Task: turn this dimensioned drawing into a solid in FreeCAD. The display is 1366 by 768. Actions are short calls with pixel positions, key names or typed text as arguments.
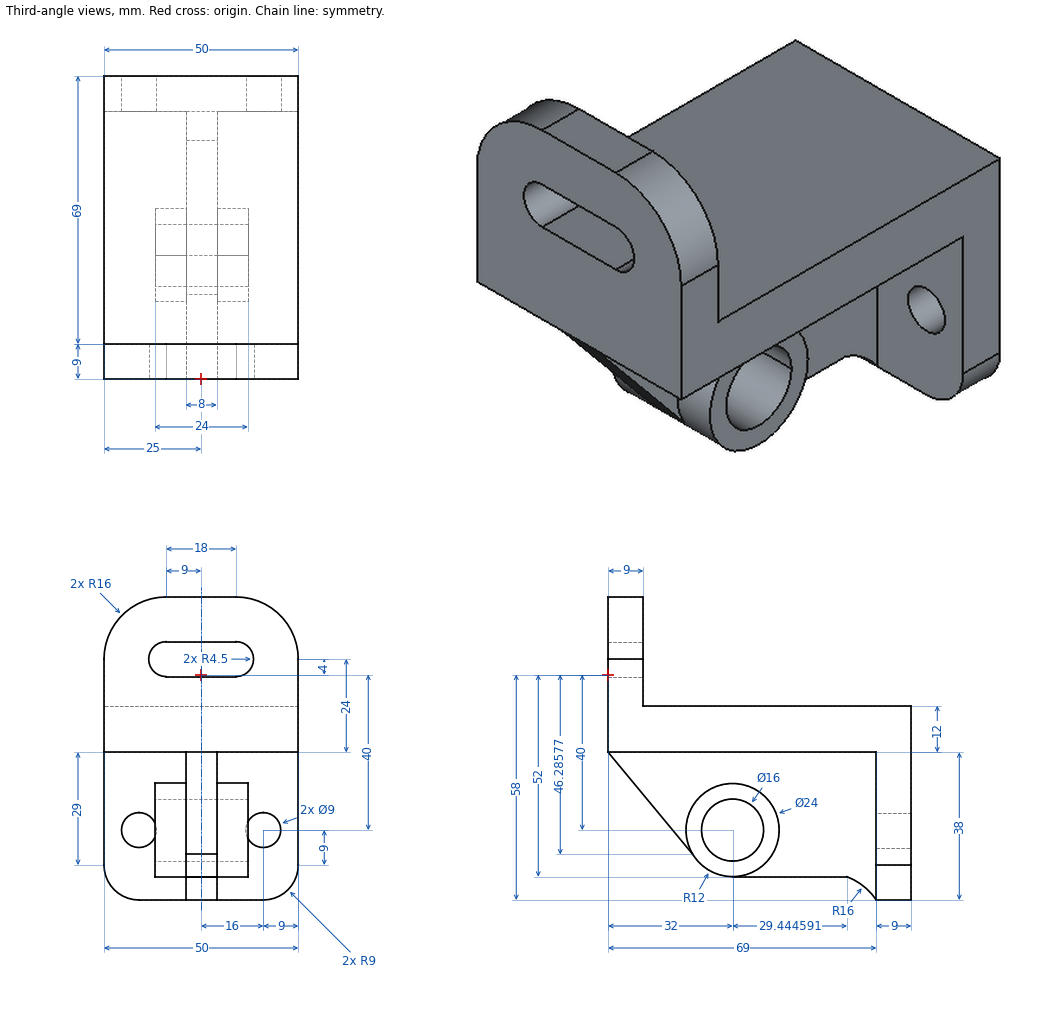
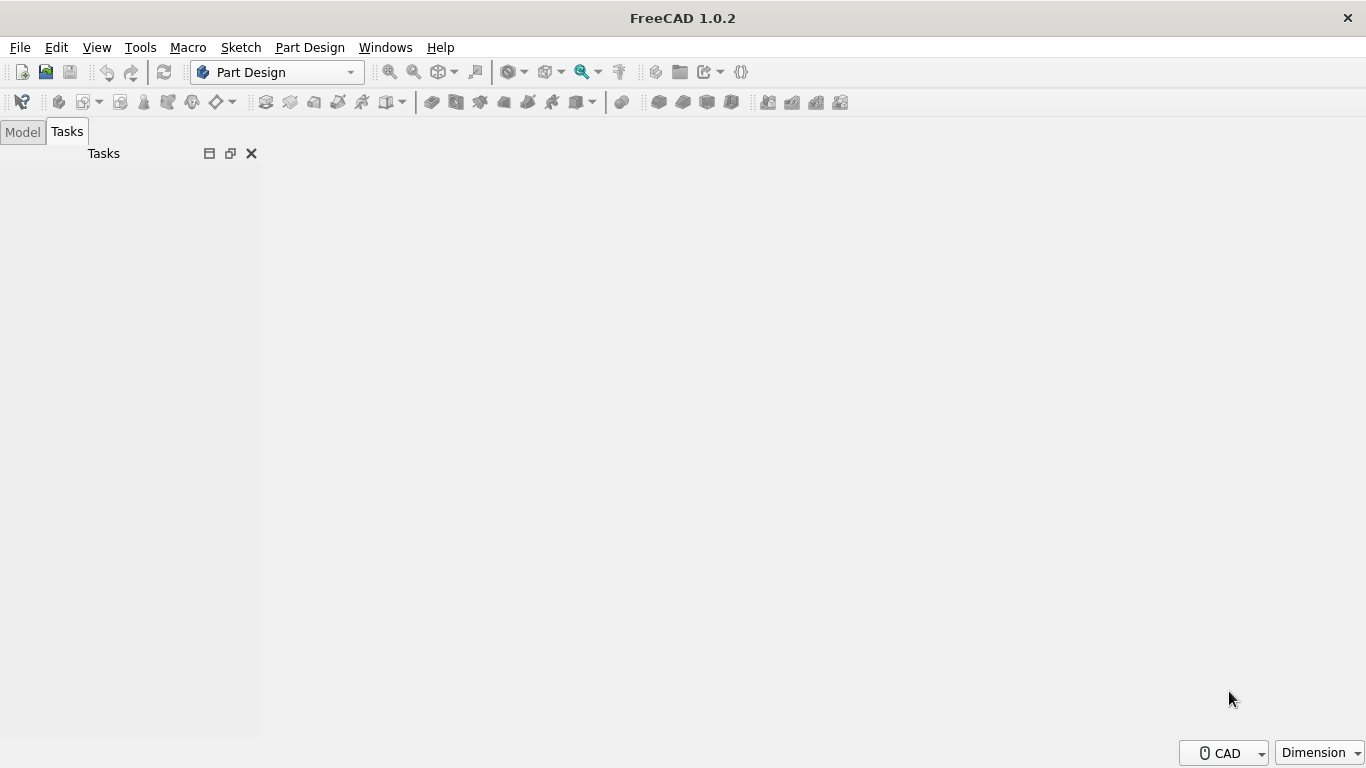
click(22, 72)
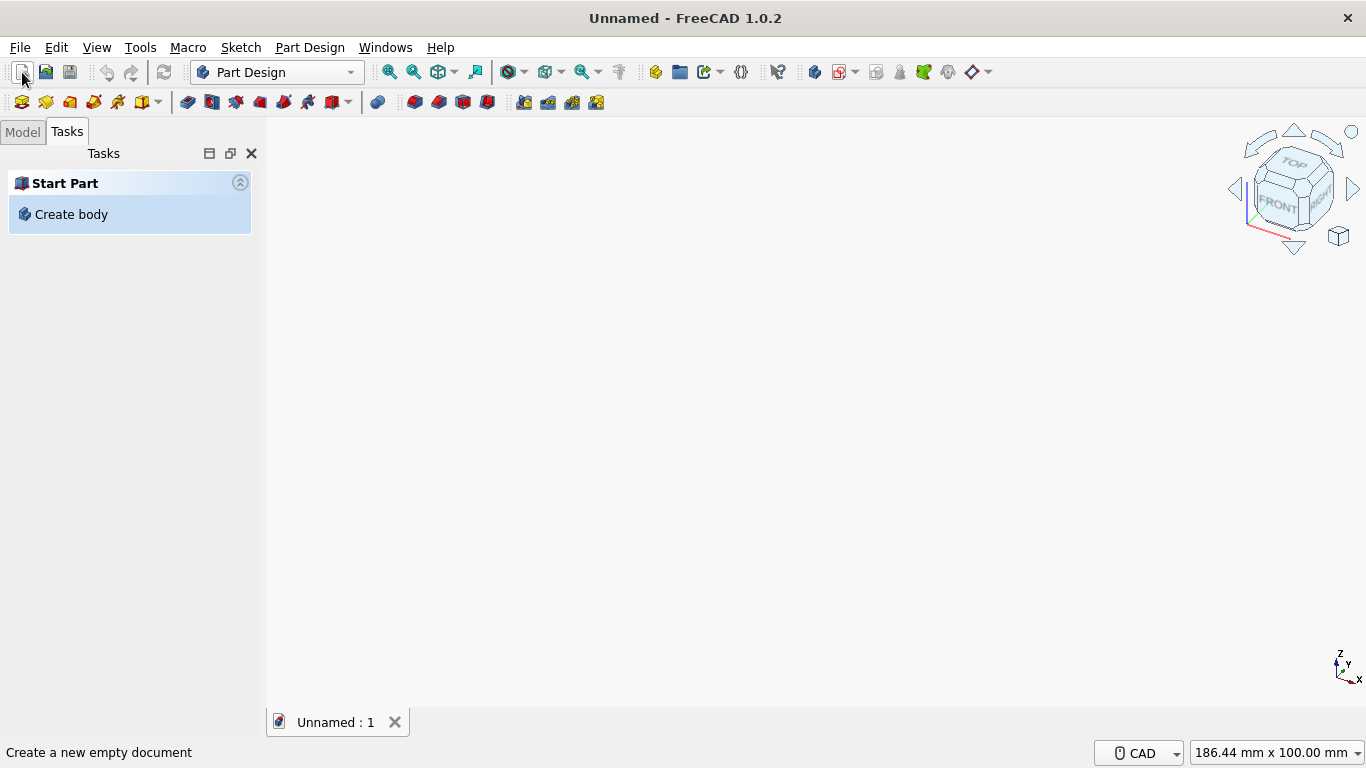
click(840, 72)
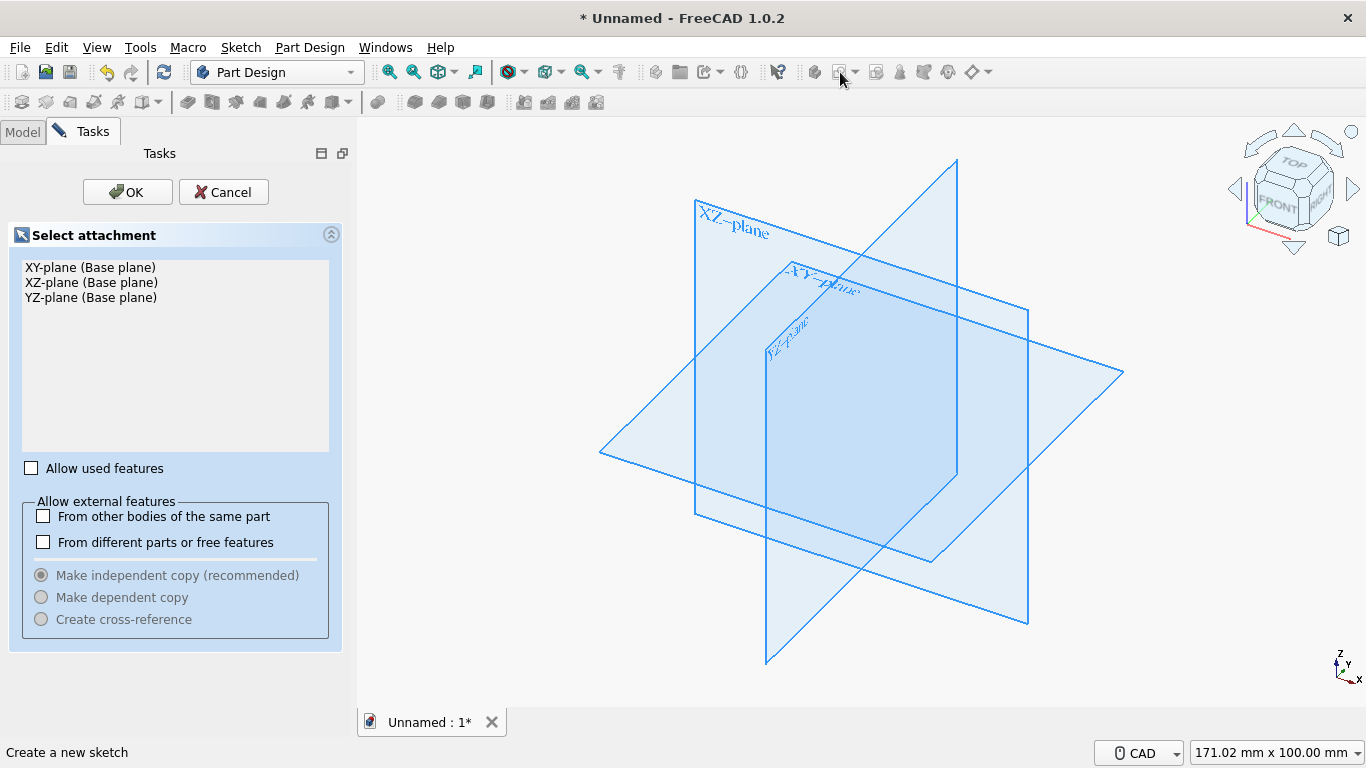
click(82, 282)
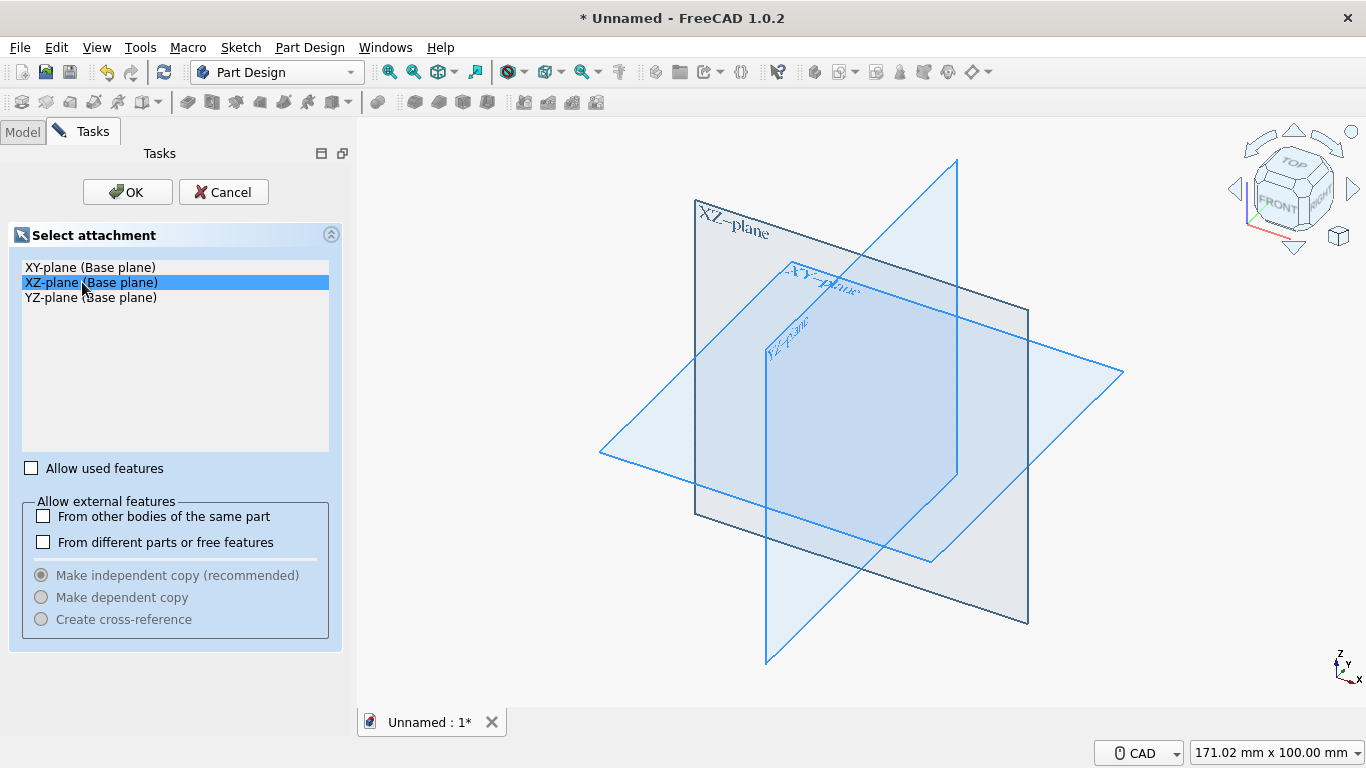
click(128, 192)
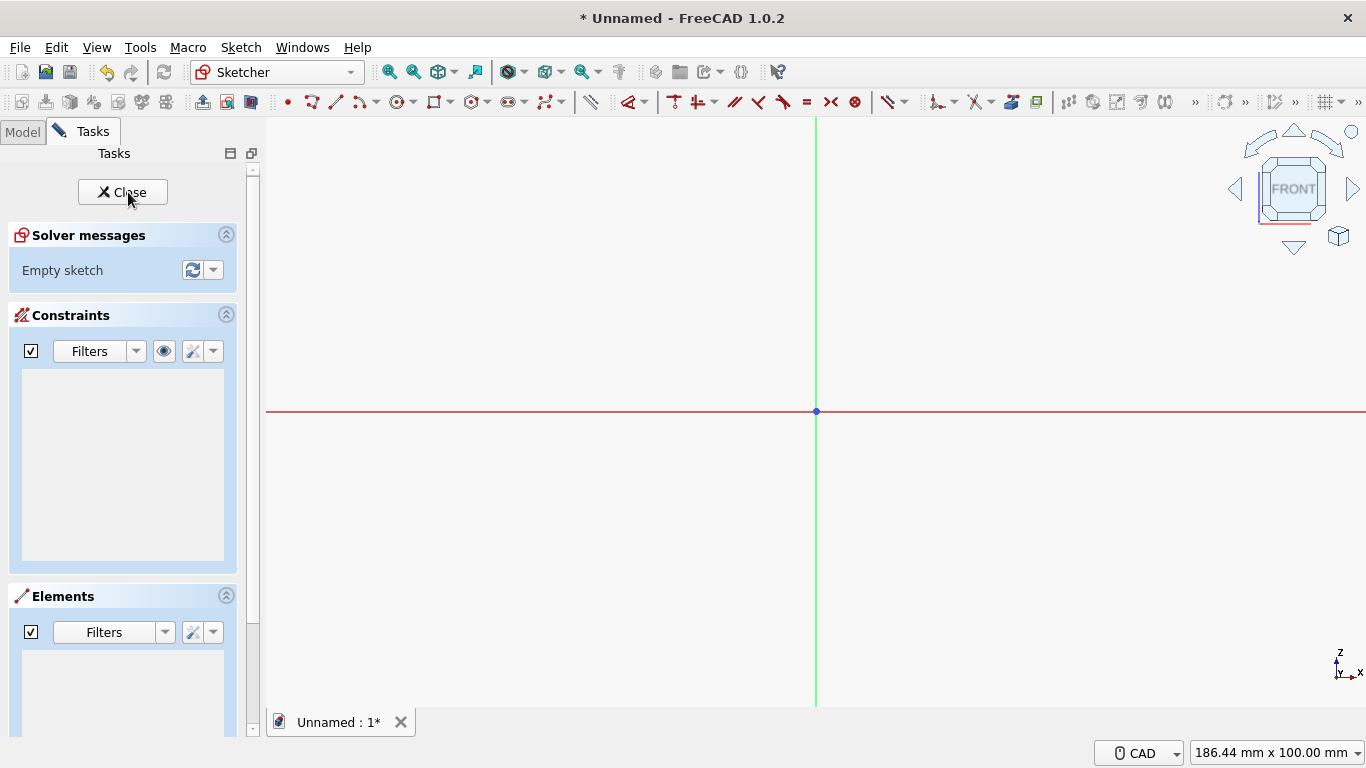
scroll(955, 412, up, 2)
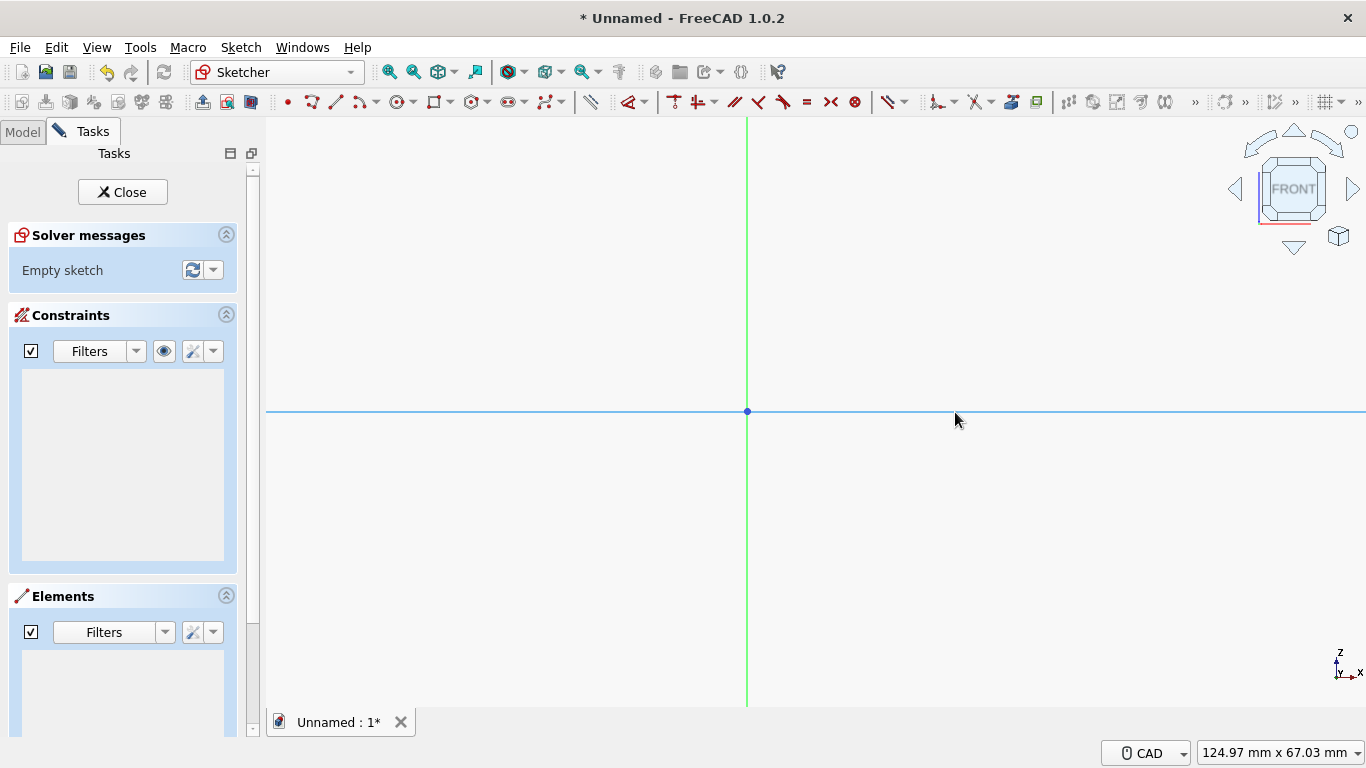
click(336, 102)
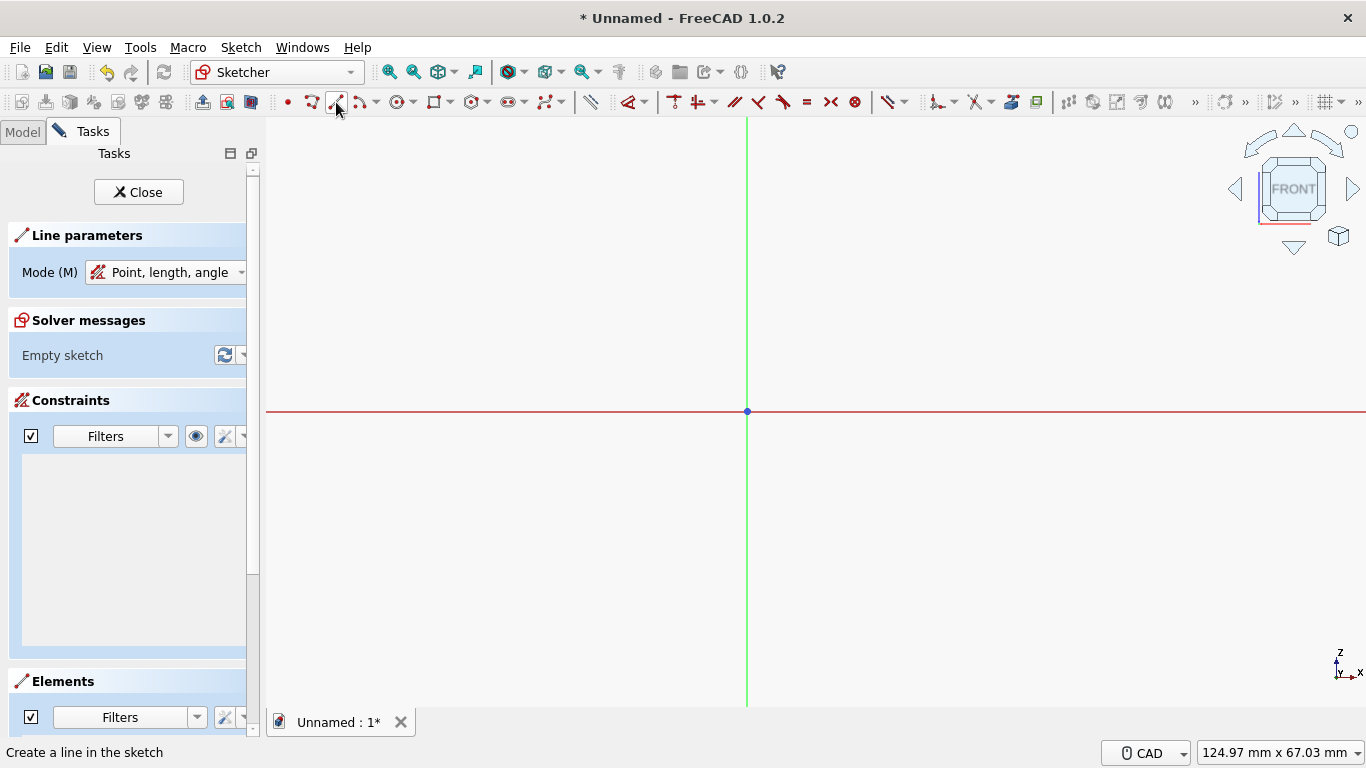
click(668, 236)
click(827, 236)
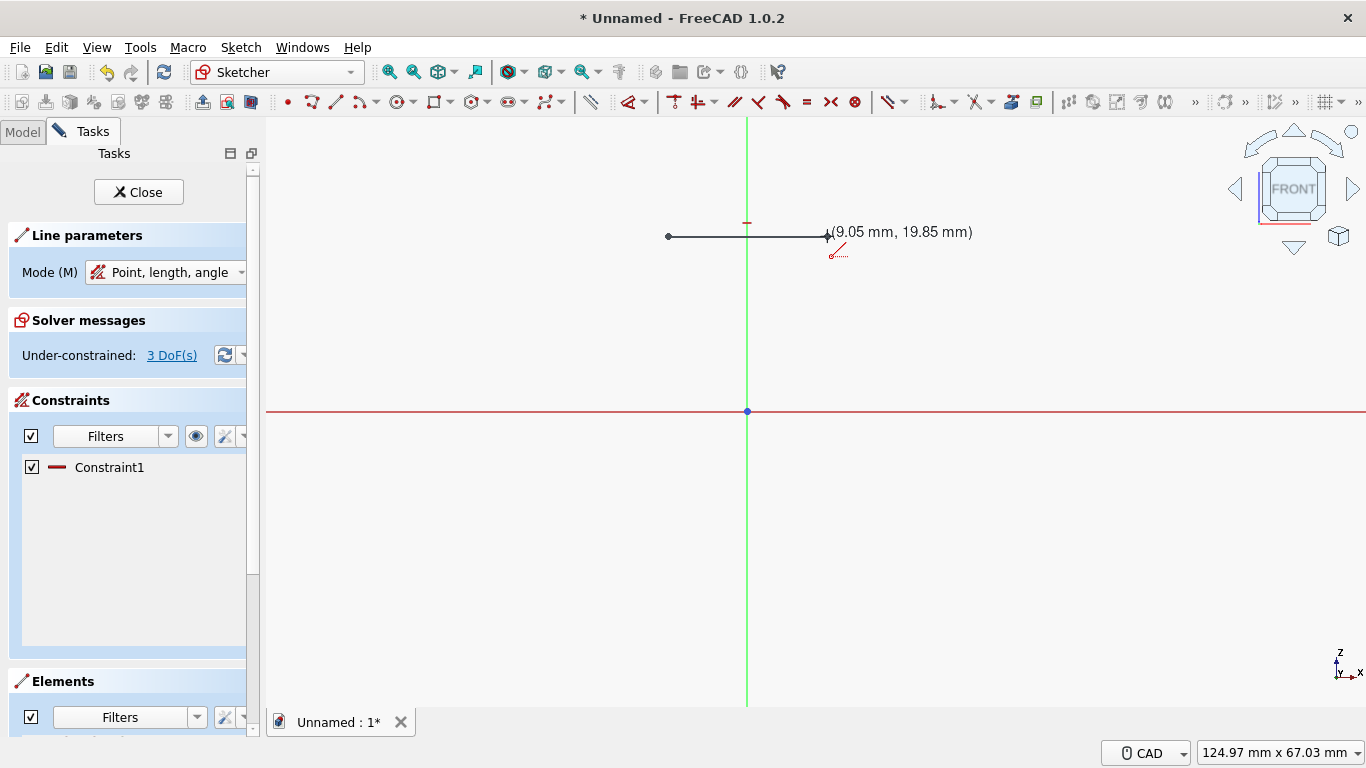
click(312, 102)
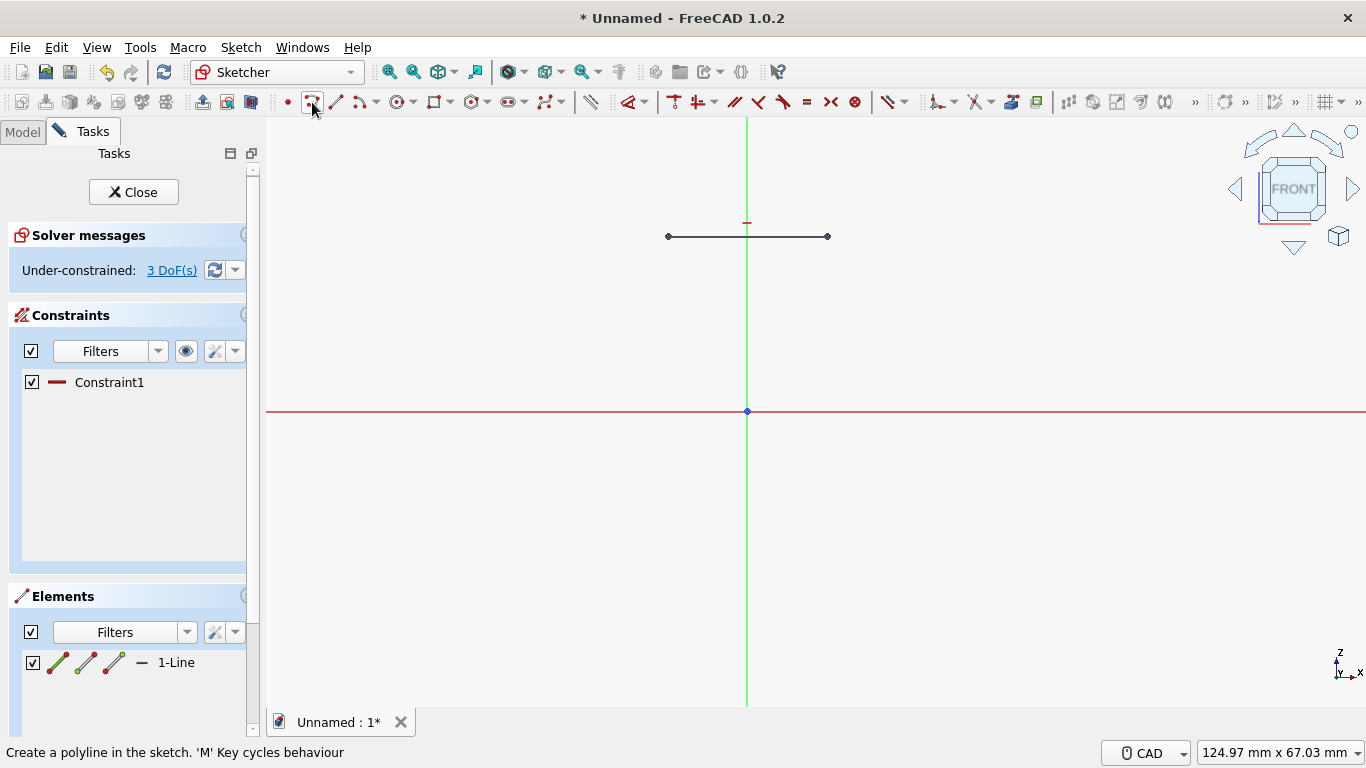
click(967, 377)
click(967, 588)
click(527, 588)
click(527, 377)
right_click(527, 377)